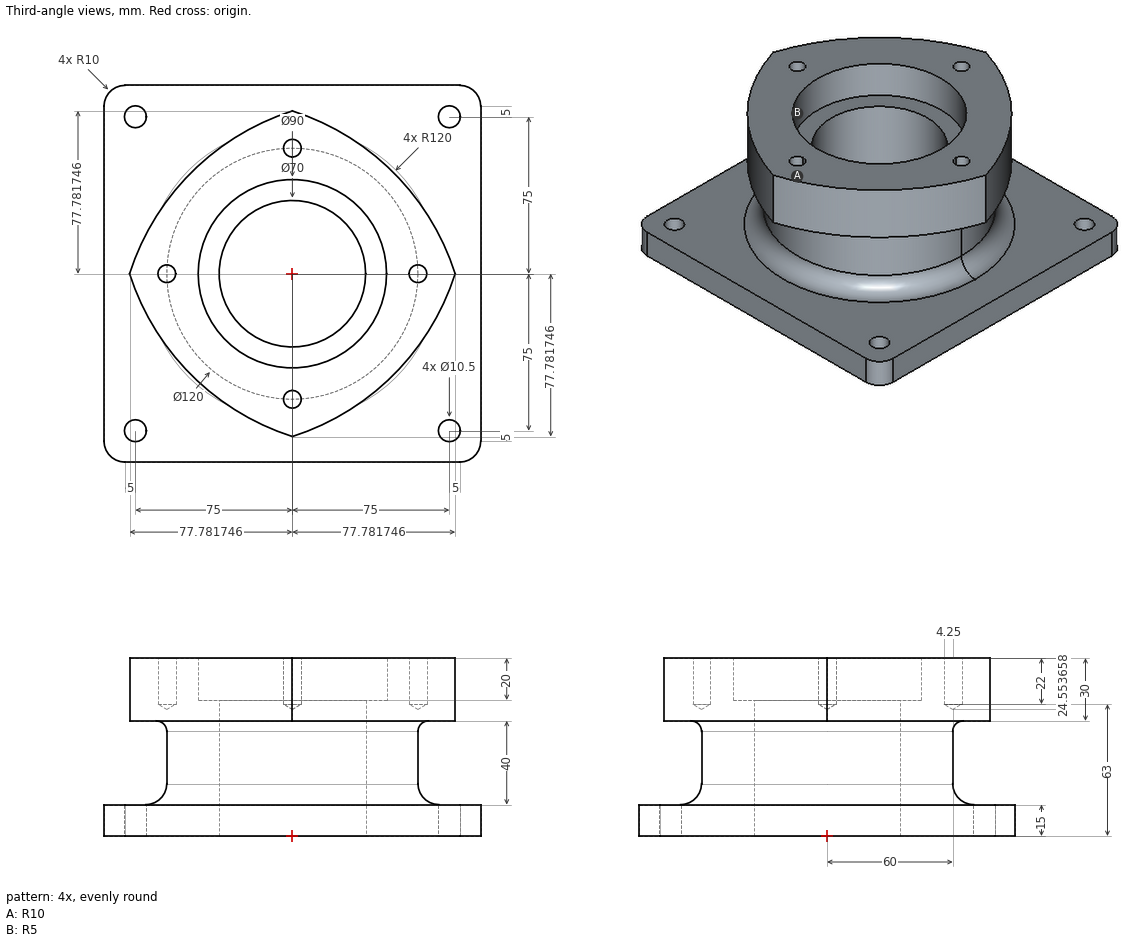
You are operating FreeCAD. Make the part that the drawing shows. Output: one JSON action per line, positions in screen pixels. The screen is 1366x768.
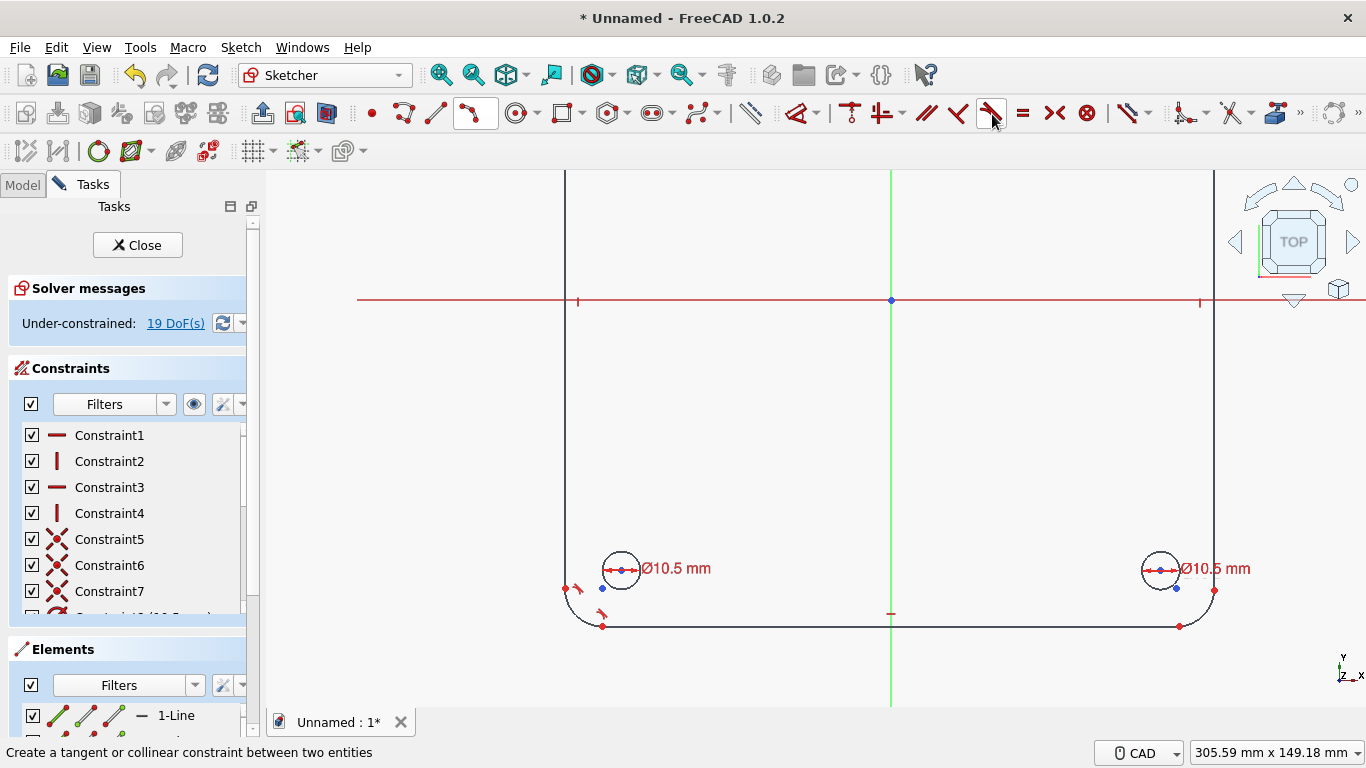
{"action": "left_click", "coordinate": [776, 627]}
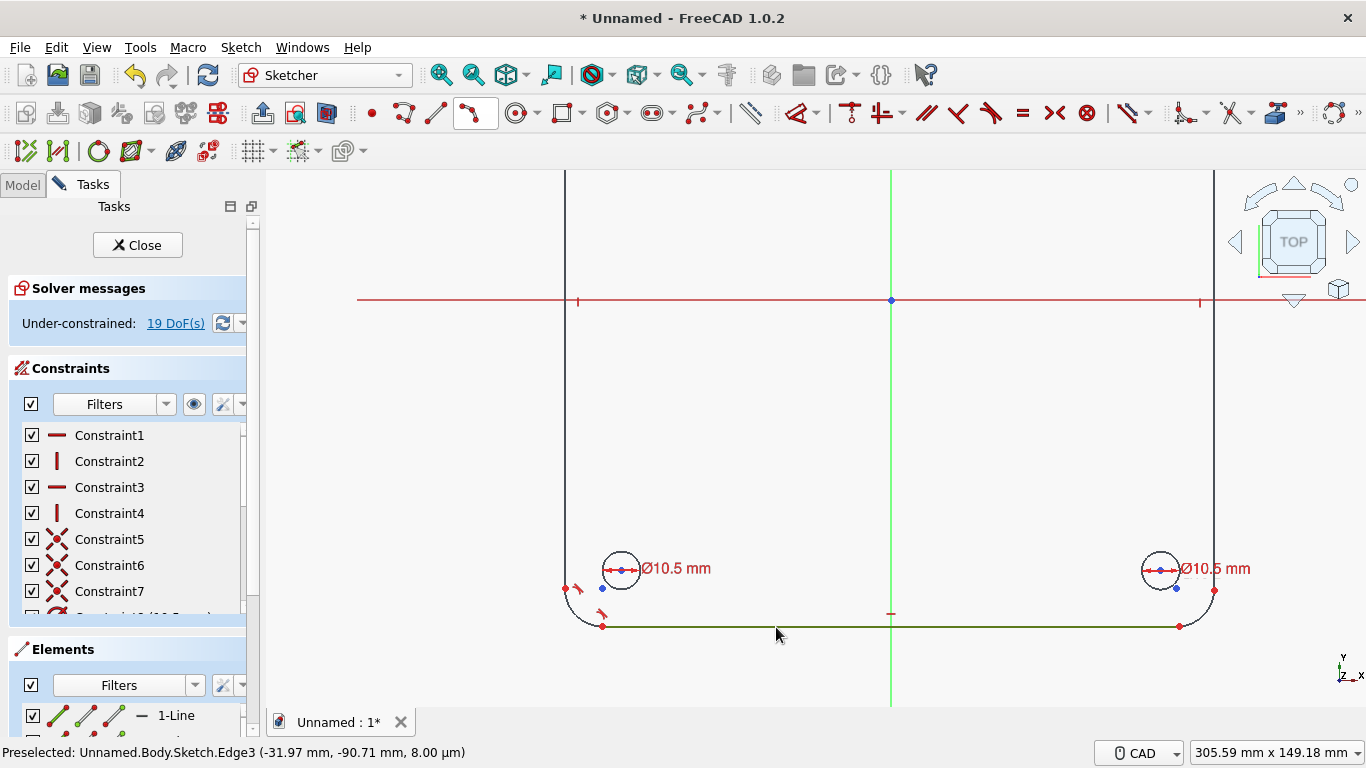
{"action": "left_click", "coordinate": [1195, 622]}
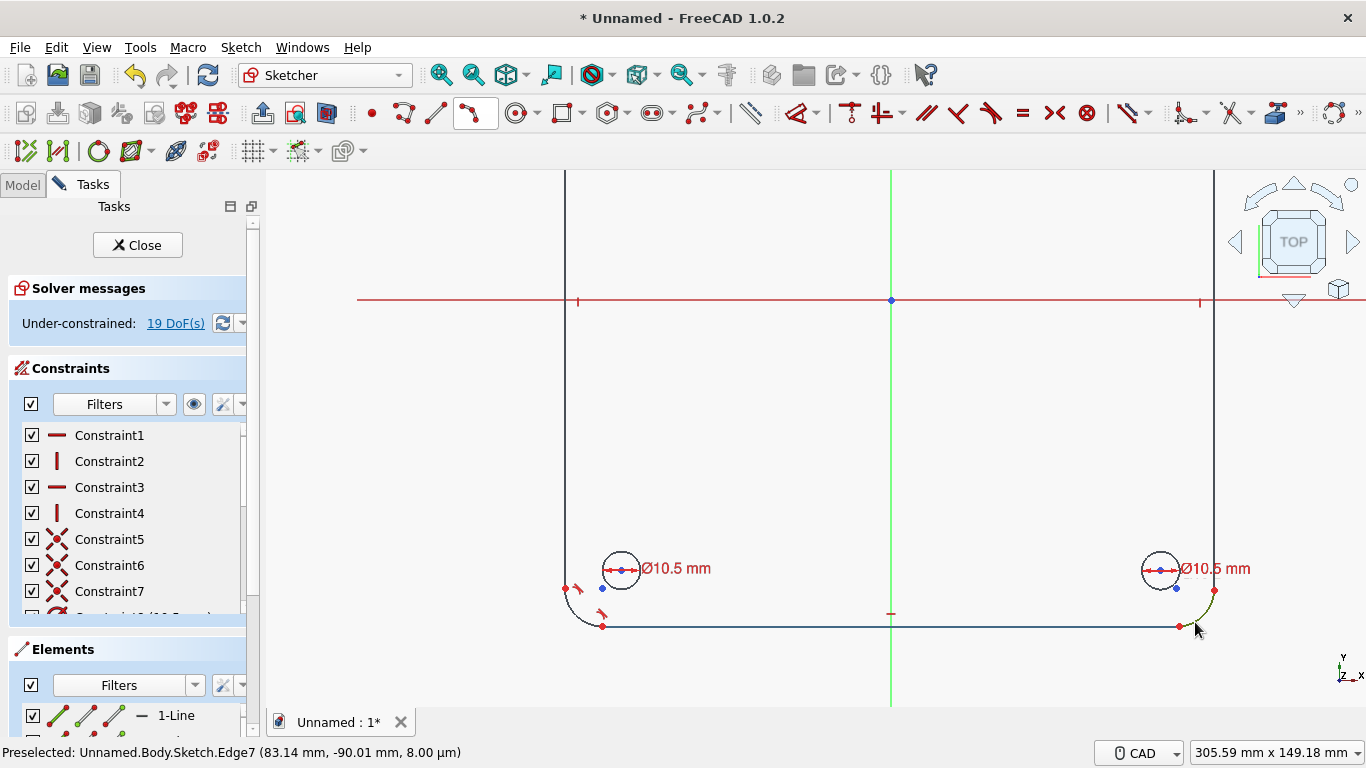
{"action": "left_click", "coordinate": [992, 114]}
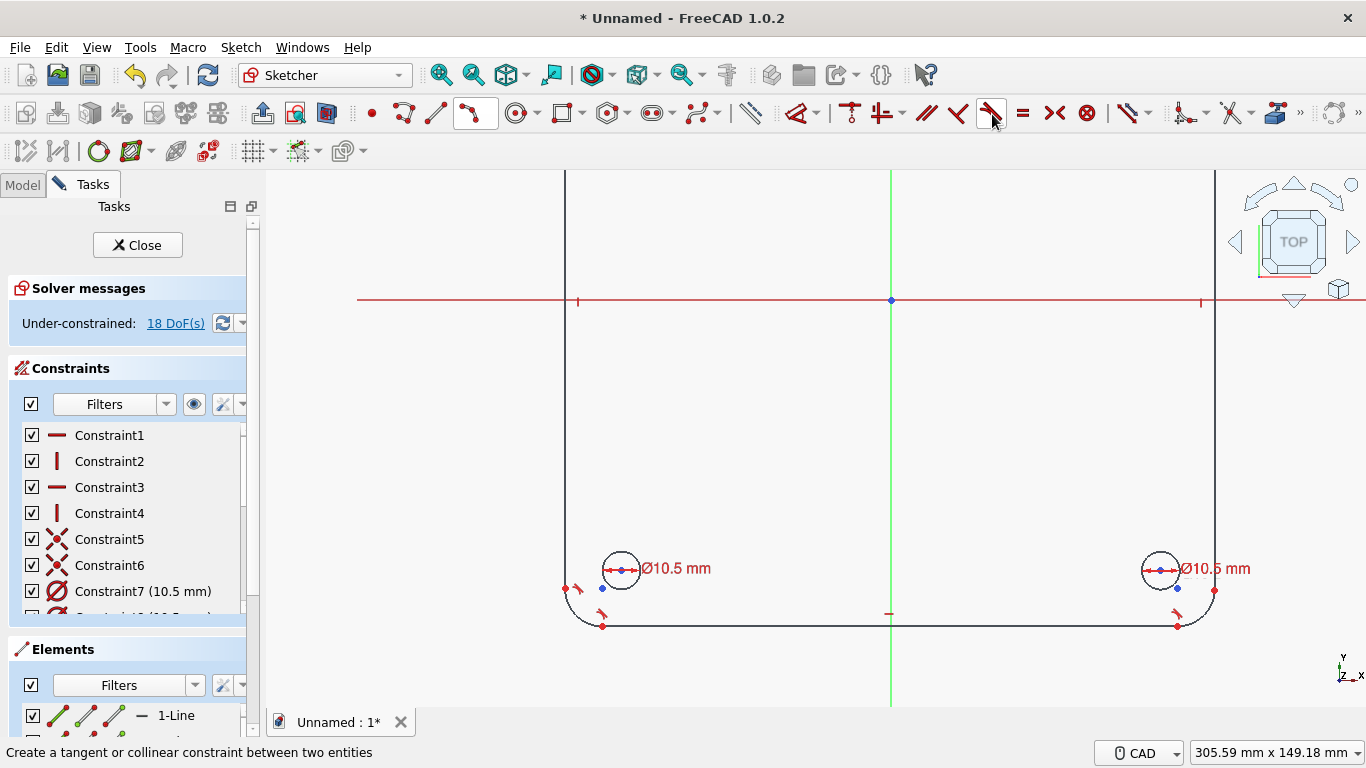
{"action": "scroll", "coordinate": [573, 607], "scroll_direction": "down", "scroll_amount": 3}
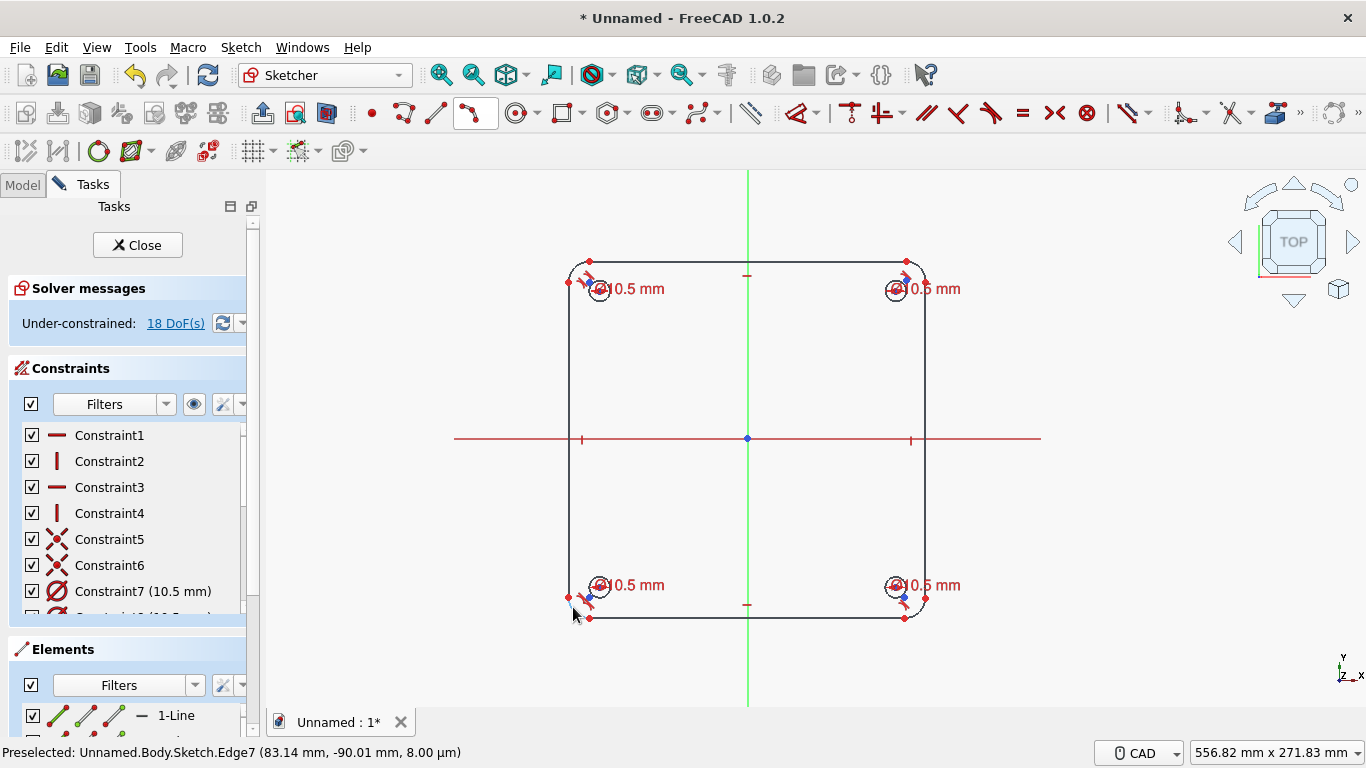
{"action": "left_click", "coordinate": [925, 503]}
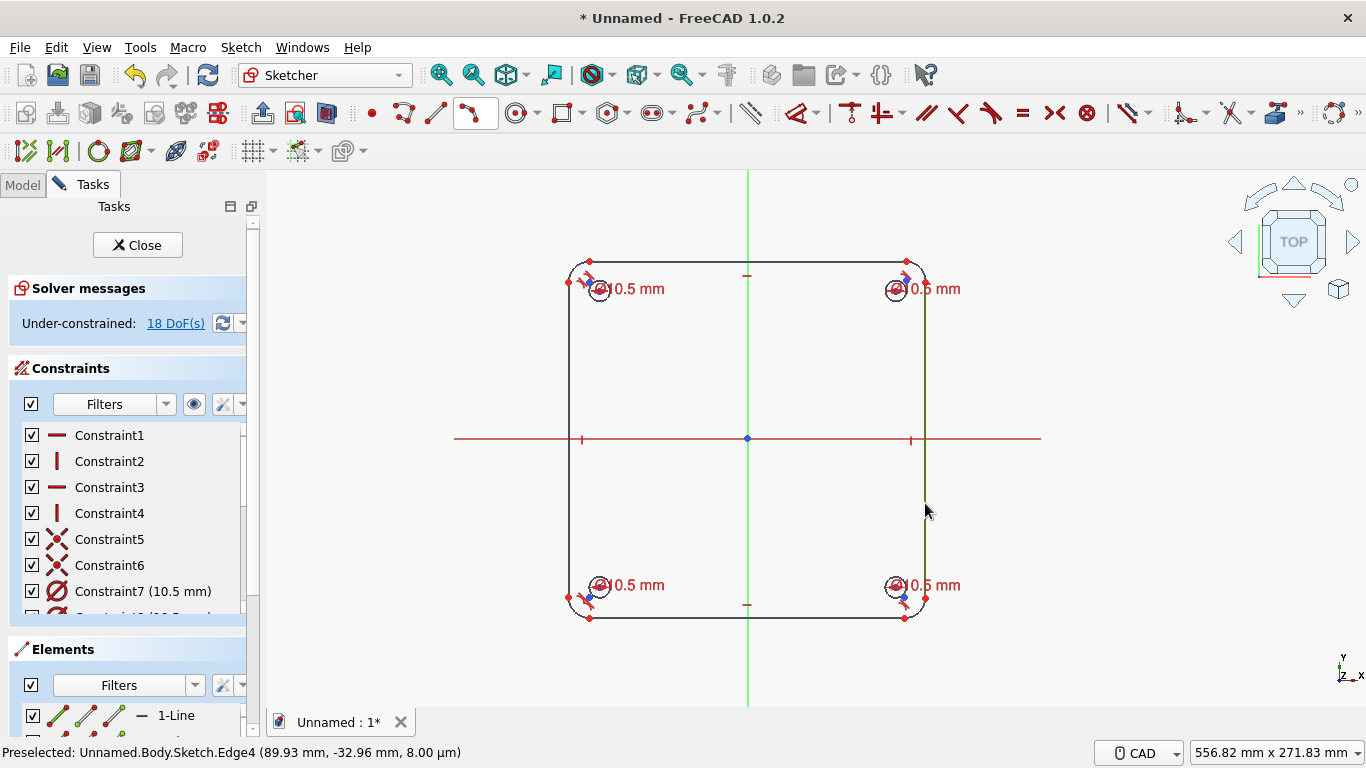
{"action": "scroll", "coordinate": [914, 616], "scroll_direction": "up", "scroll_amount": 2}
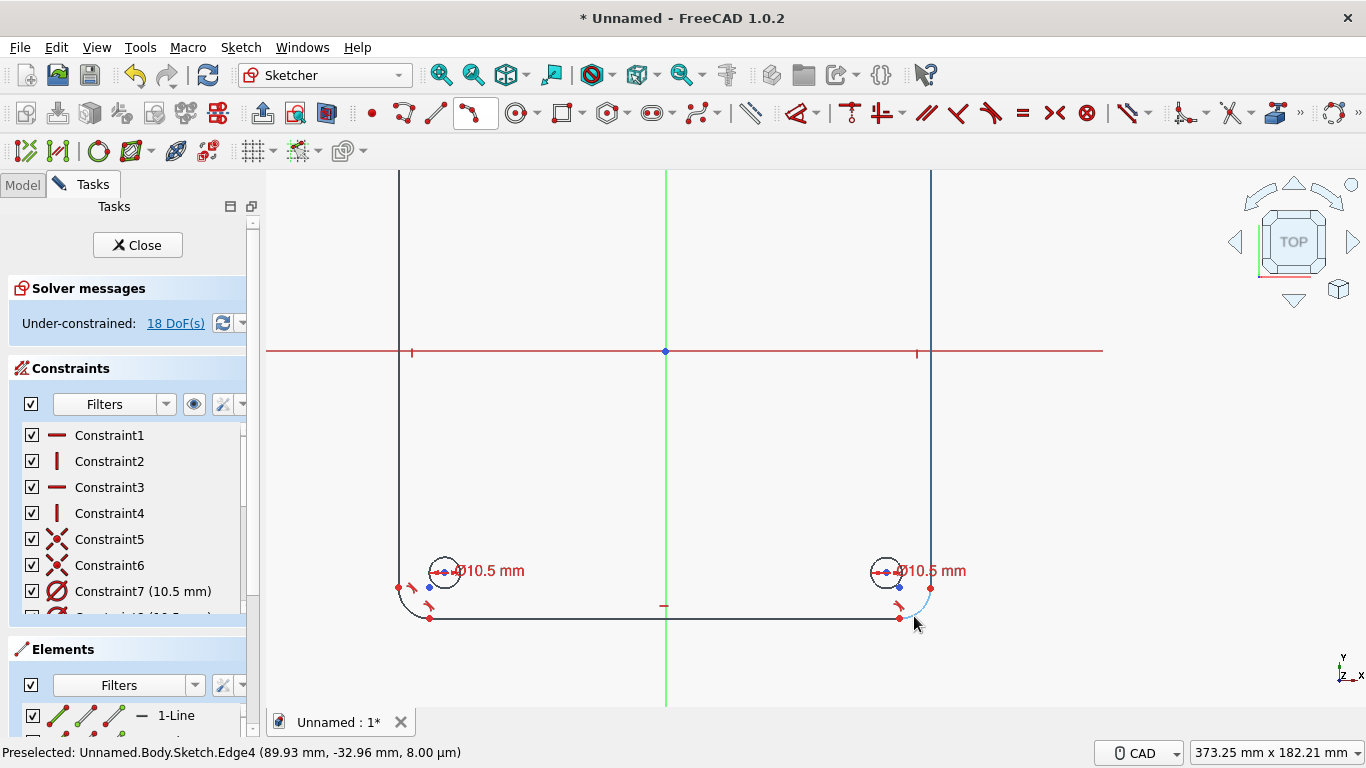
{"action": "left_click", "coordinate": [913, 615]}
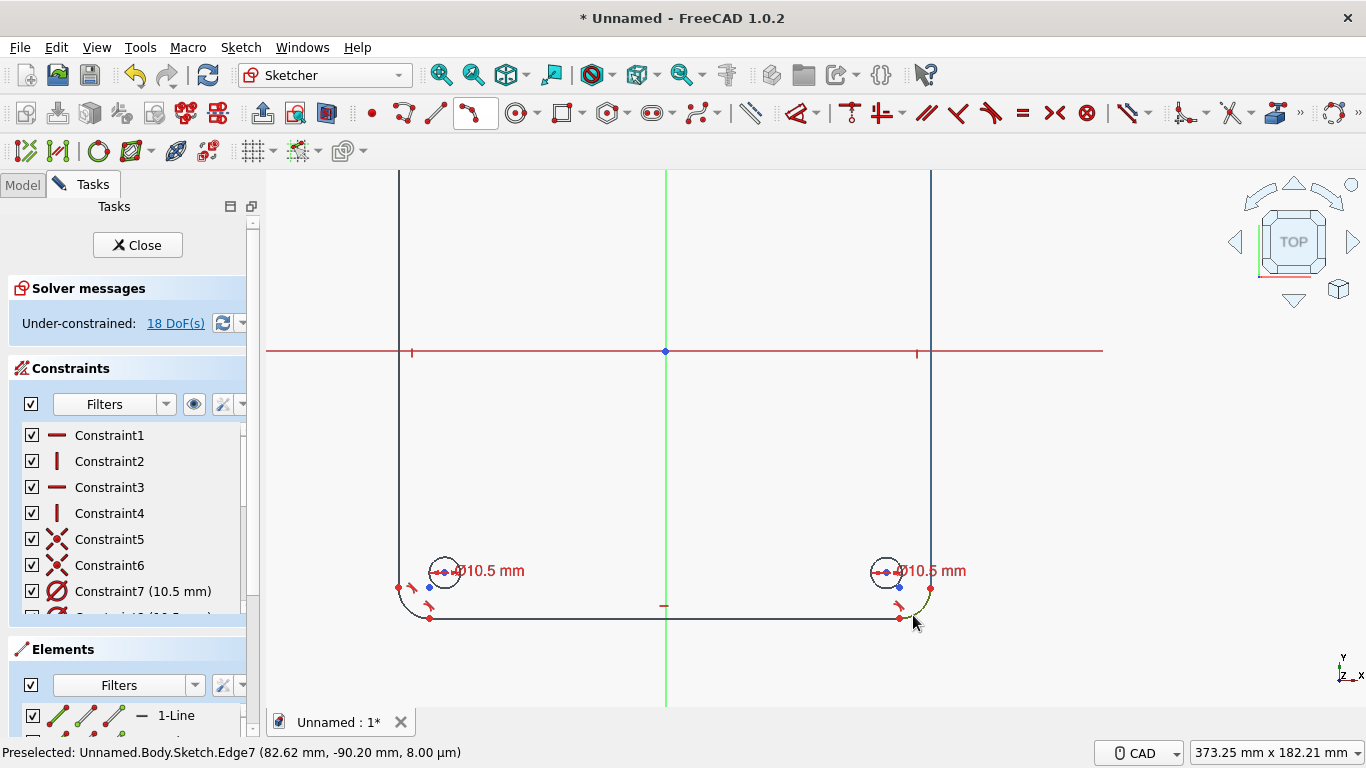
{"action": "left_click", "coordinate": [992, 114]}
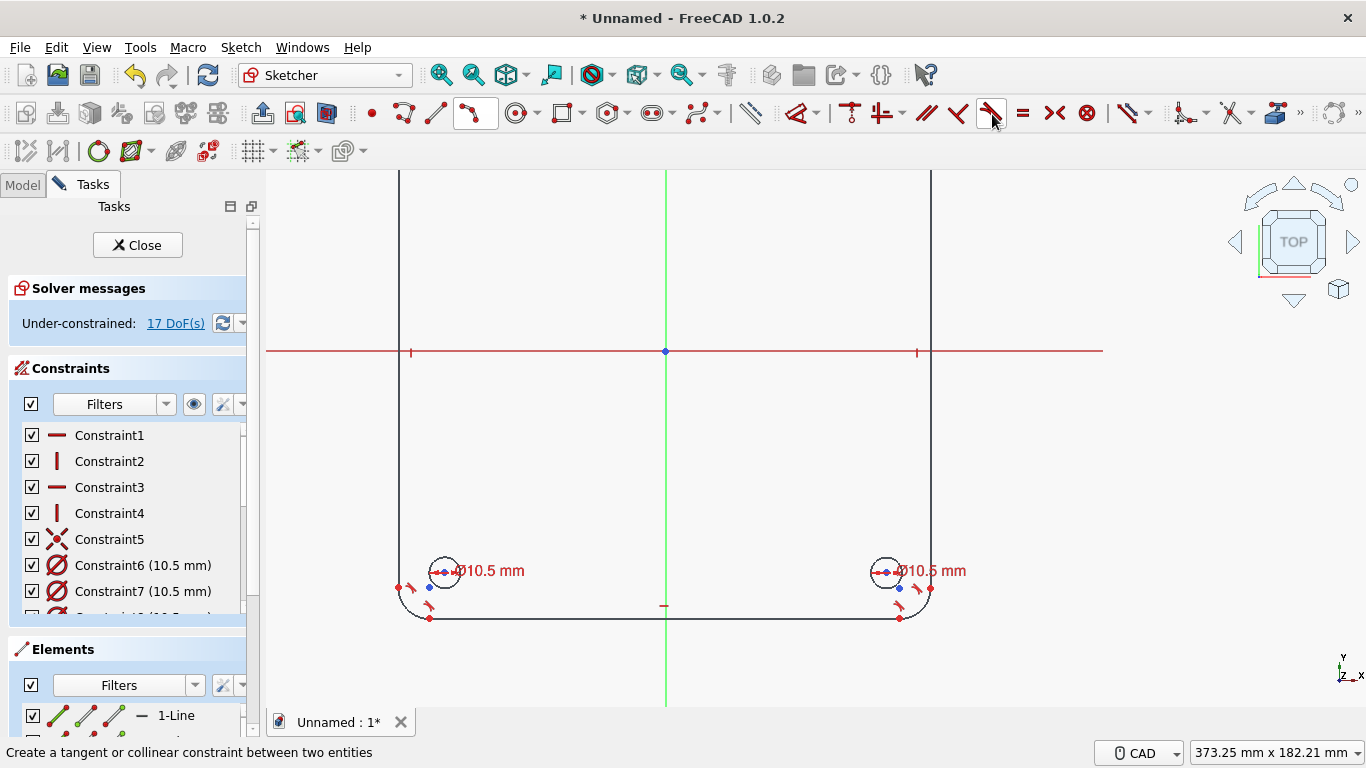
{"action": "left_click", "coordinate": [931, 447]}